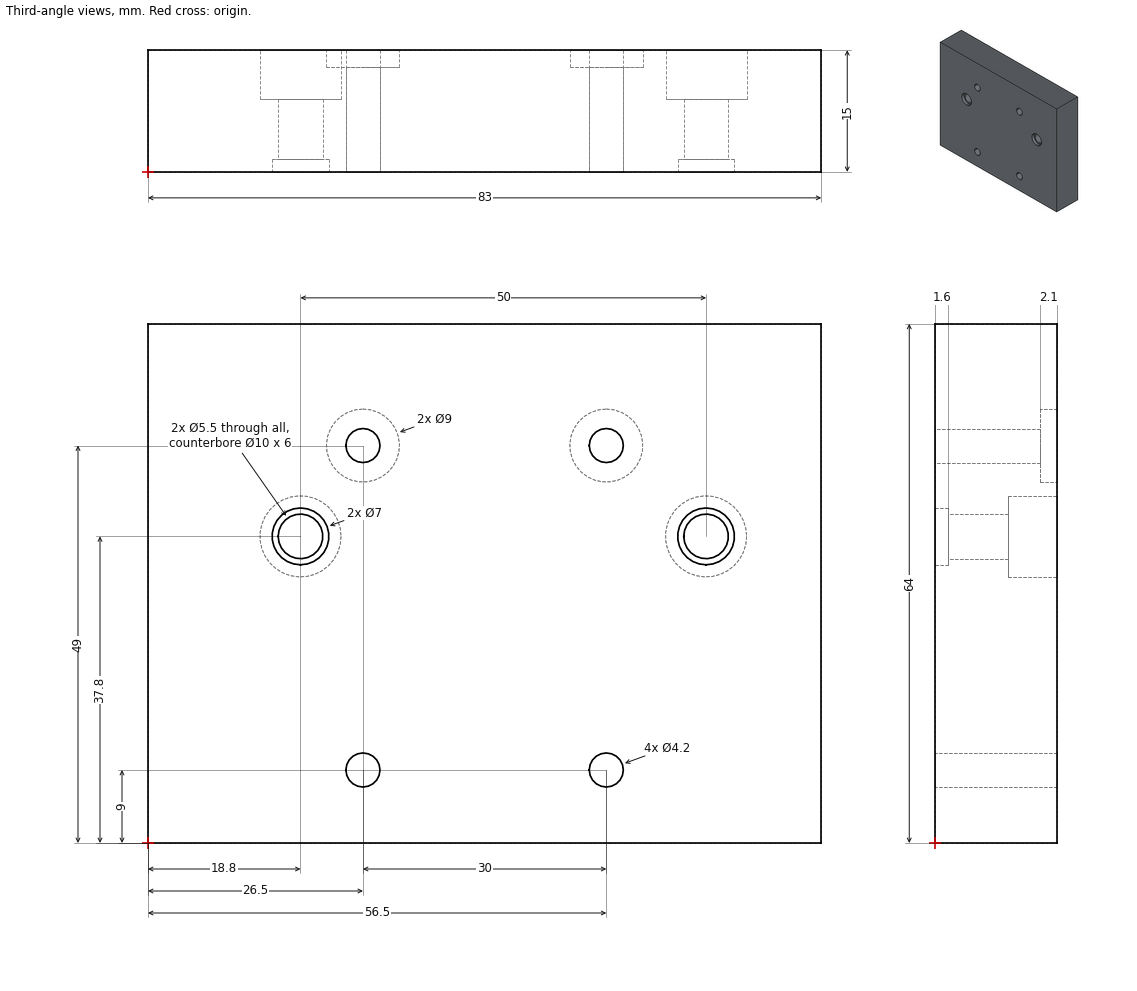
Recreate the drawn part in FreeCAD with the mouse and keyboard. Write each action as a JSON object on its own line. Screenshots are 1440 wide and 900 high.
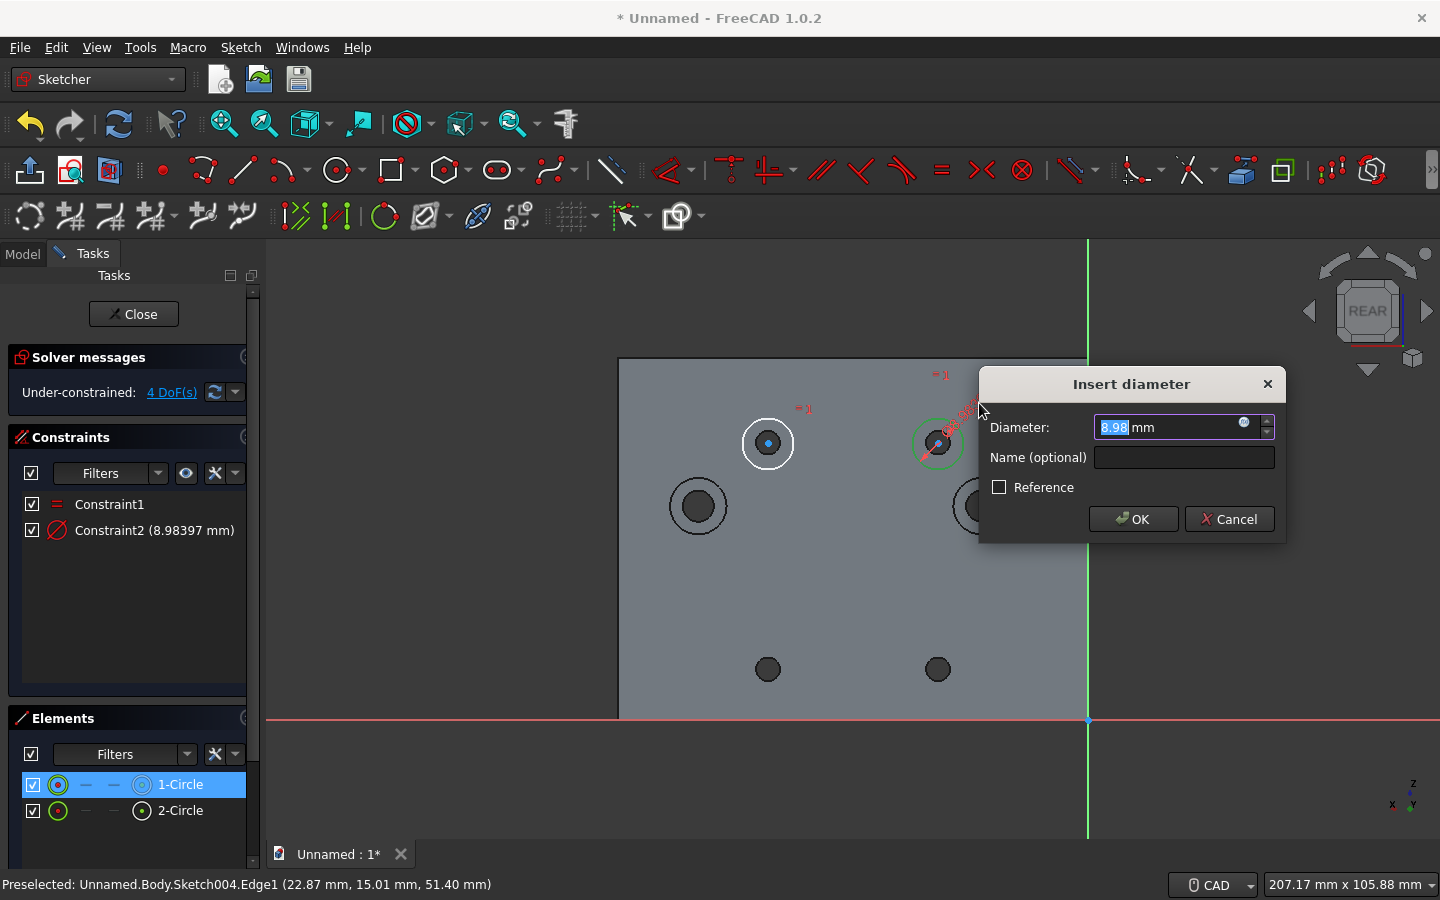
{"action": "type", "text": "9"}
{"action": "key", "text": "Return"}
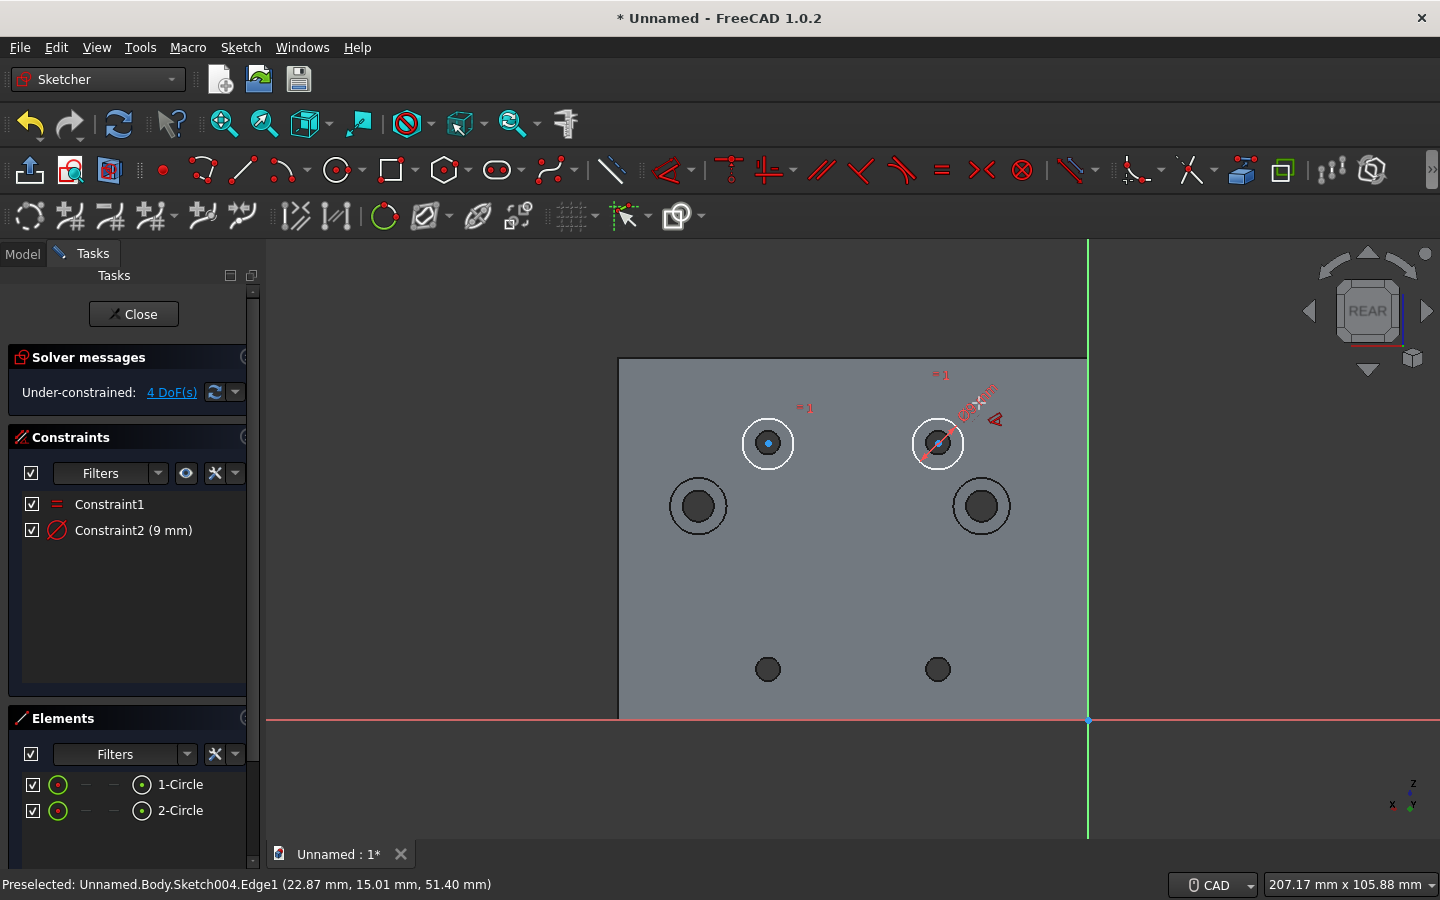
{"action": "left_click", "coordinate": [938, 444]}
{"action": "left_click", "coordinate": [1122, 582]}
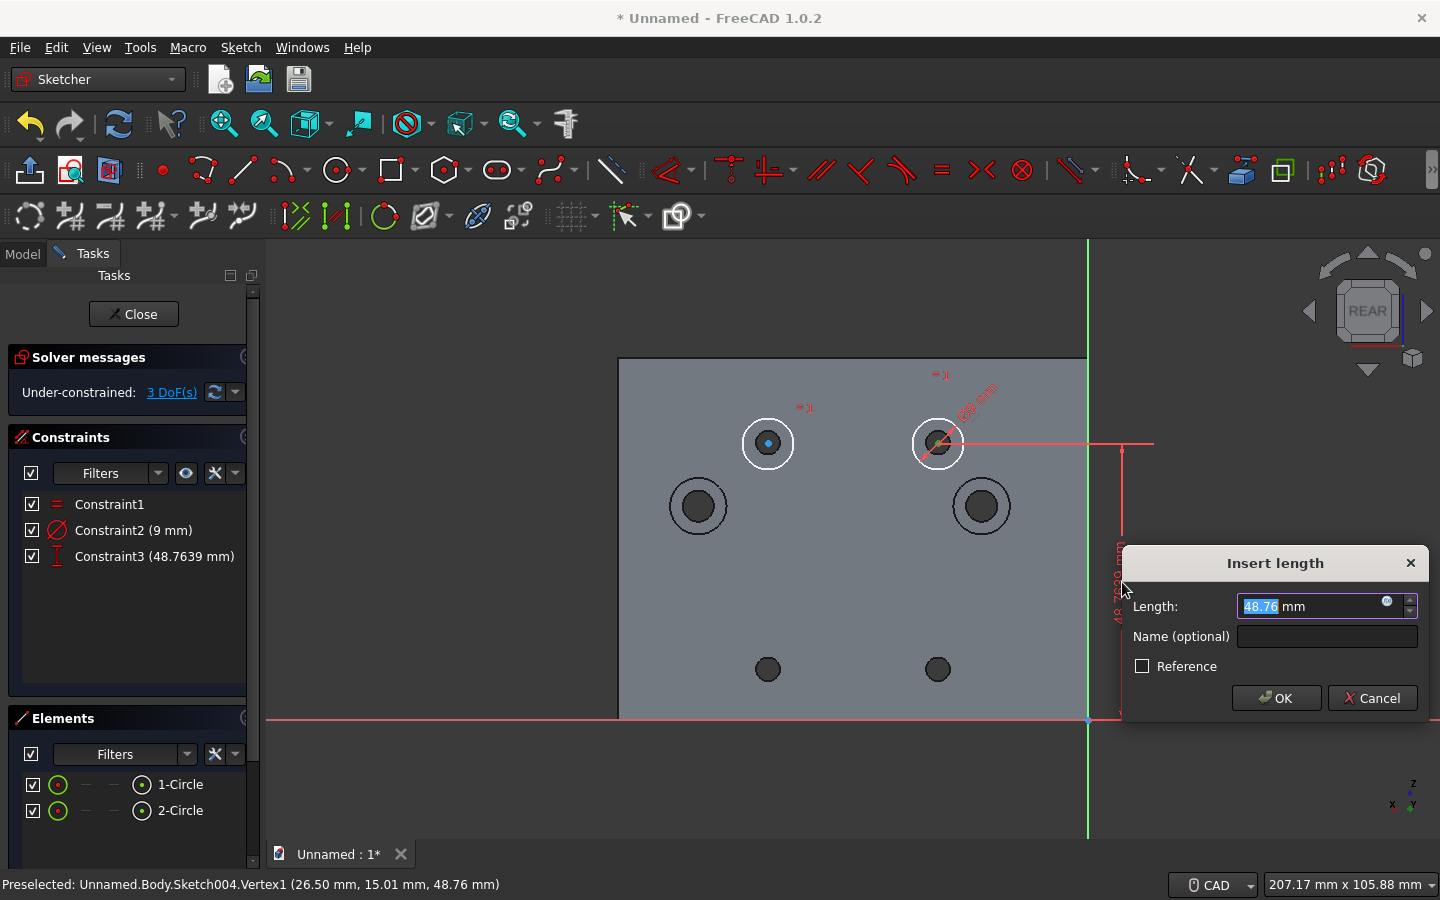
{"action": "type", "text": "49"}
{"action": "key", "text": "Return"}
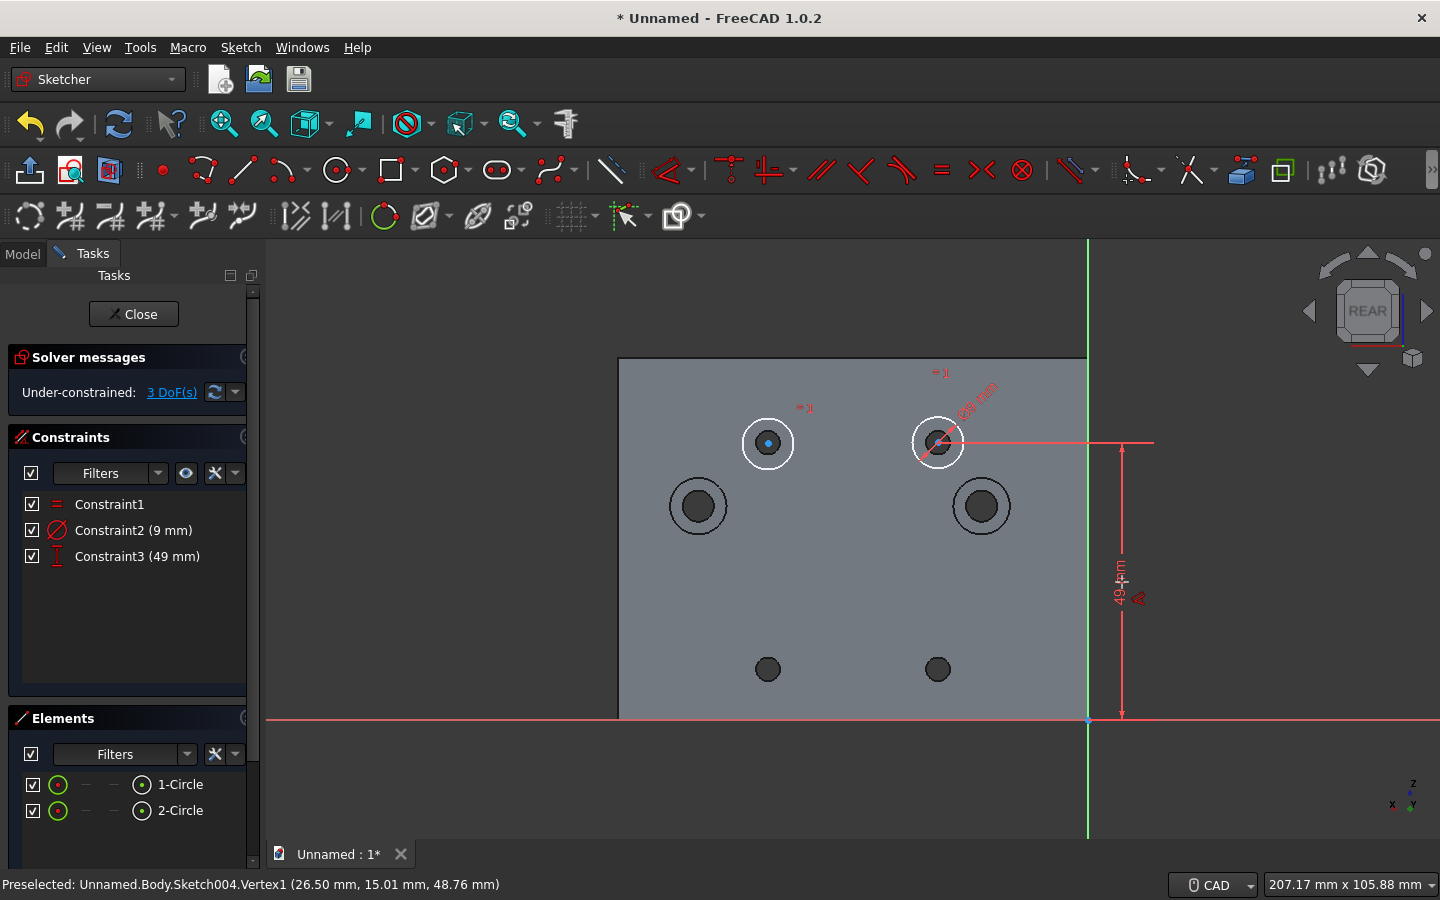
{"action": "left_click", "coordinate": [768, 444]}
{"action": "left_click", "coordinate": [1122, 519]}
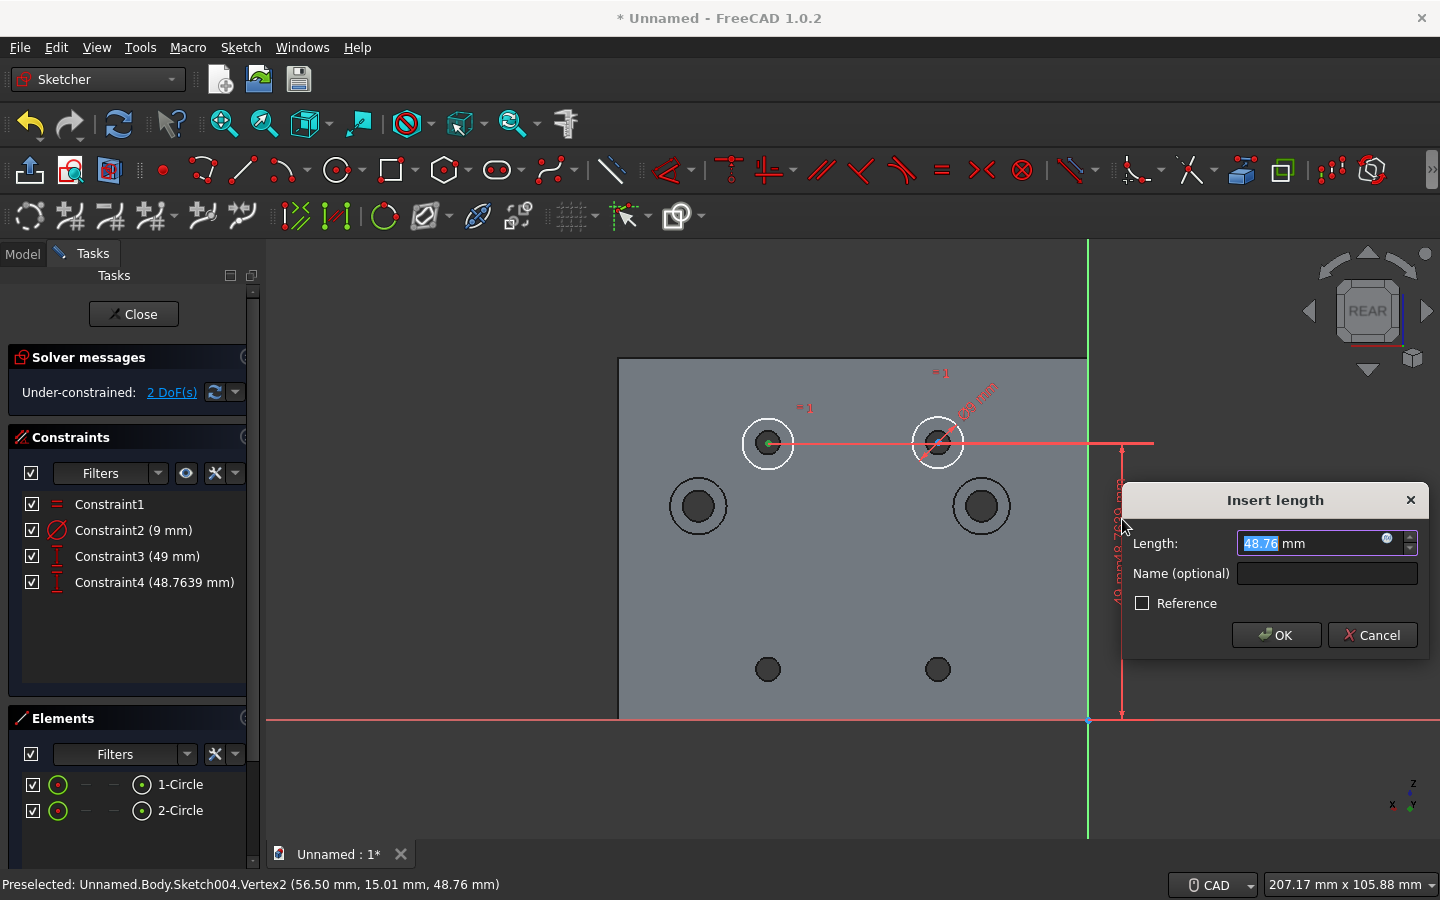
{"action": "type", "text": "49"}
{"action": "key", "text": "Return"}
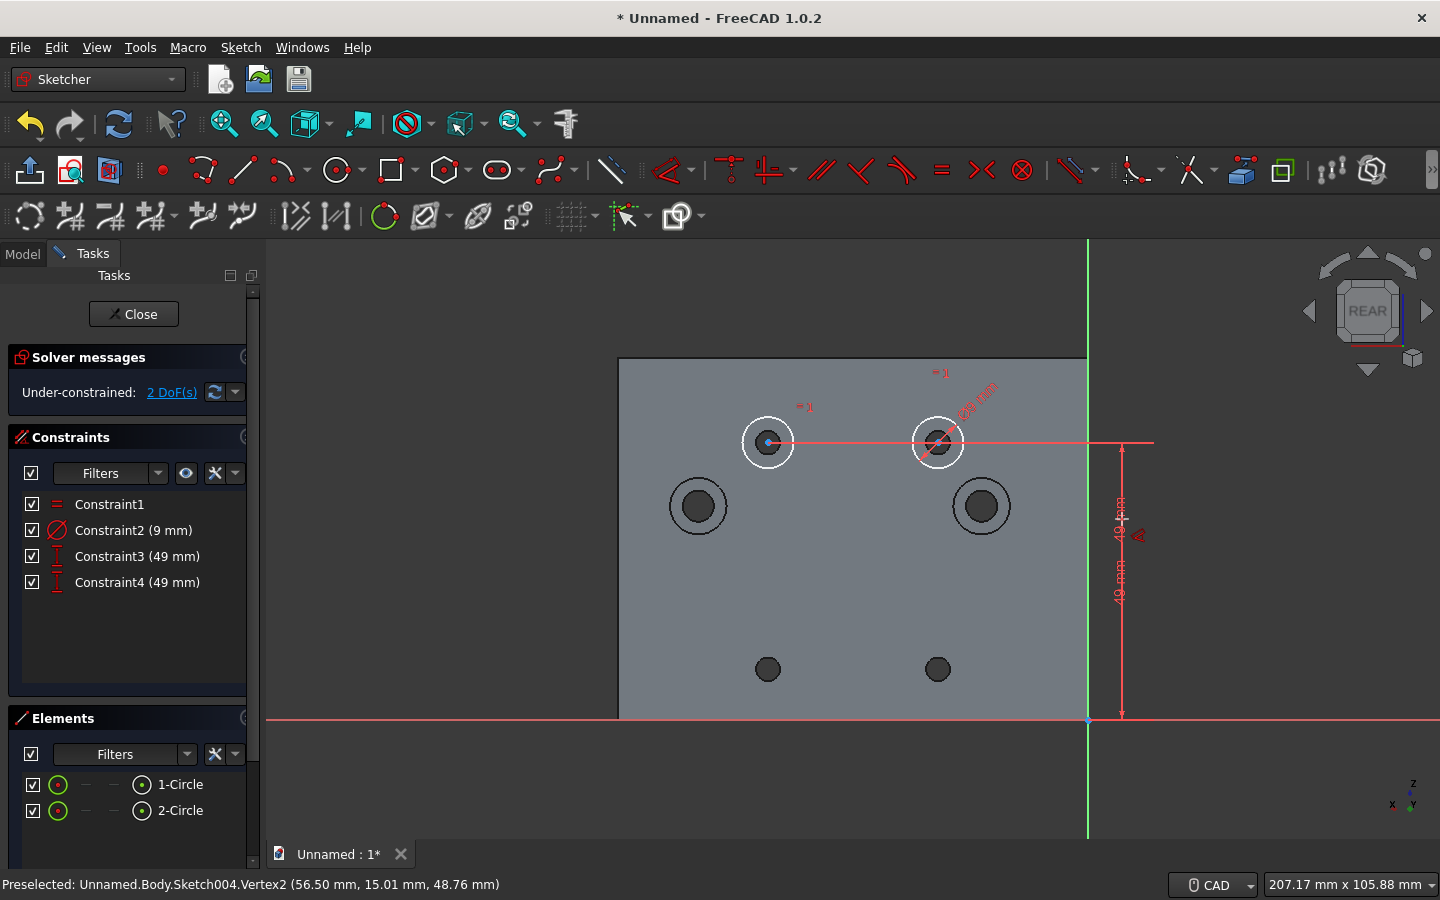
{"action": "left_click", "coordinate": [938, 443]}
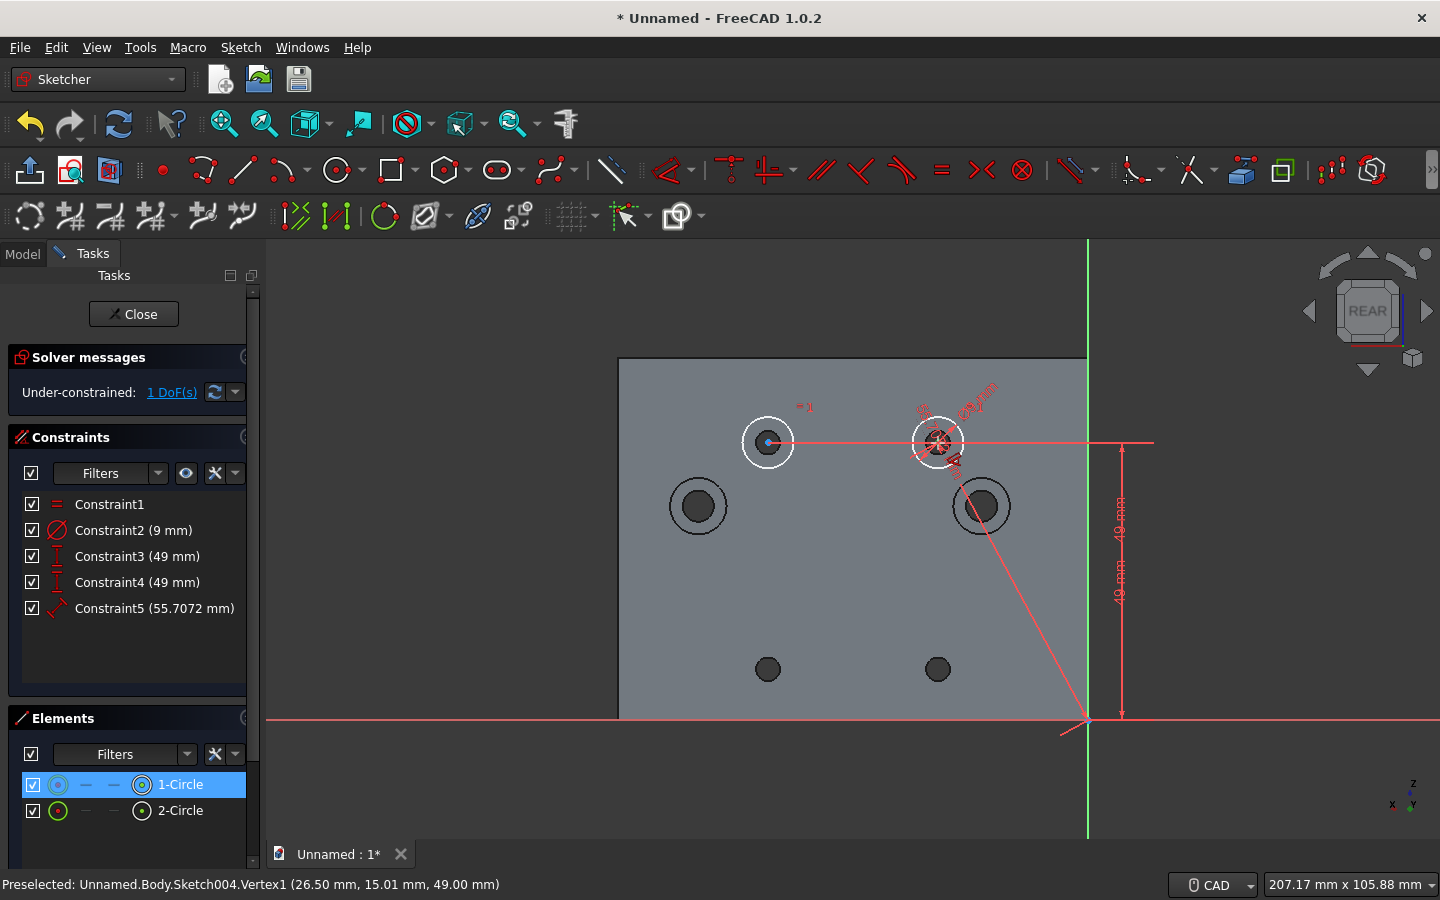
{"action": "left_click", "coordinate": [768, 443]}
{"action": "left_click", "coordinate": [853, 409]}